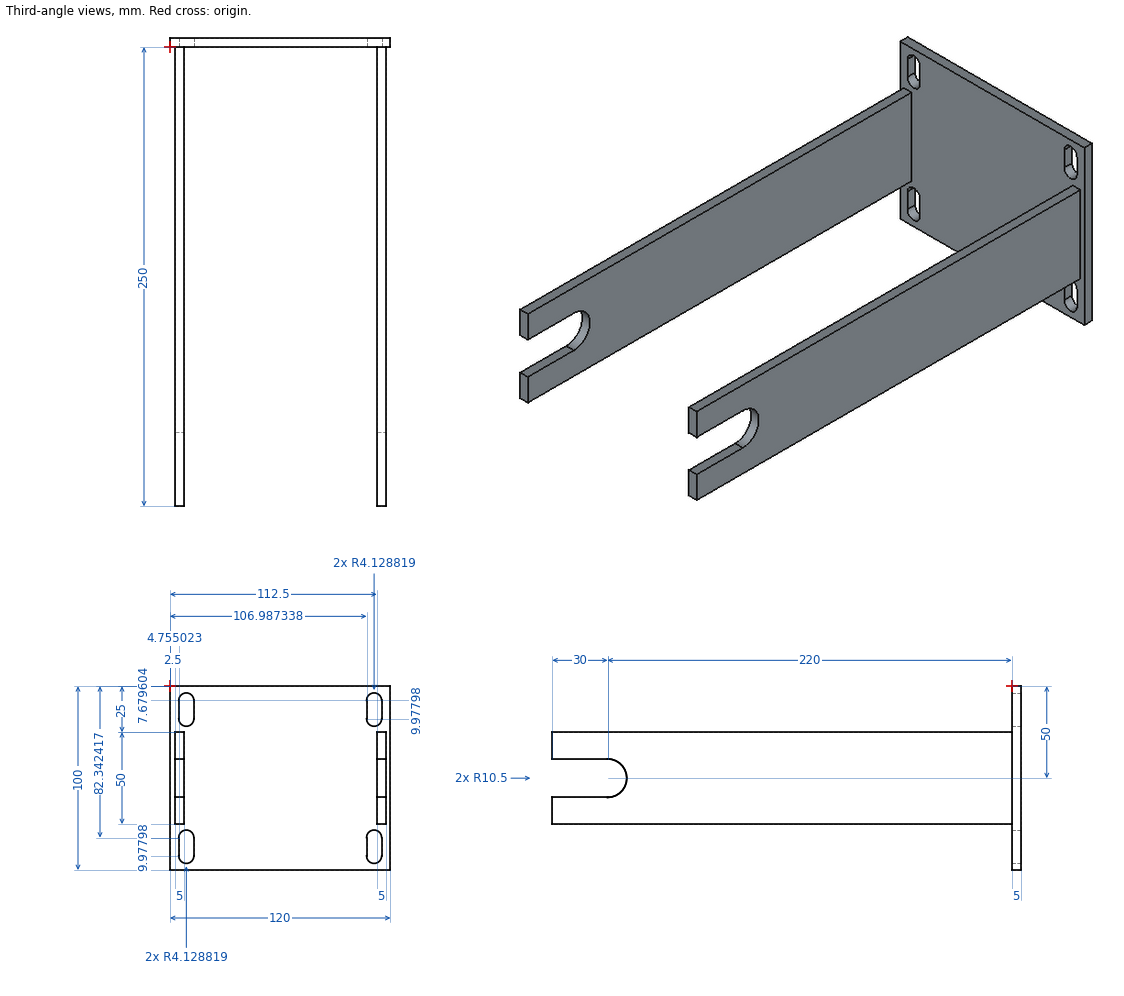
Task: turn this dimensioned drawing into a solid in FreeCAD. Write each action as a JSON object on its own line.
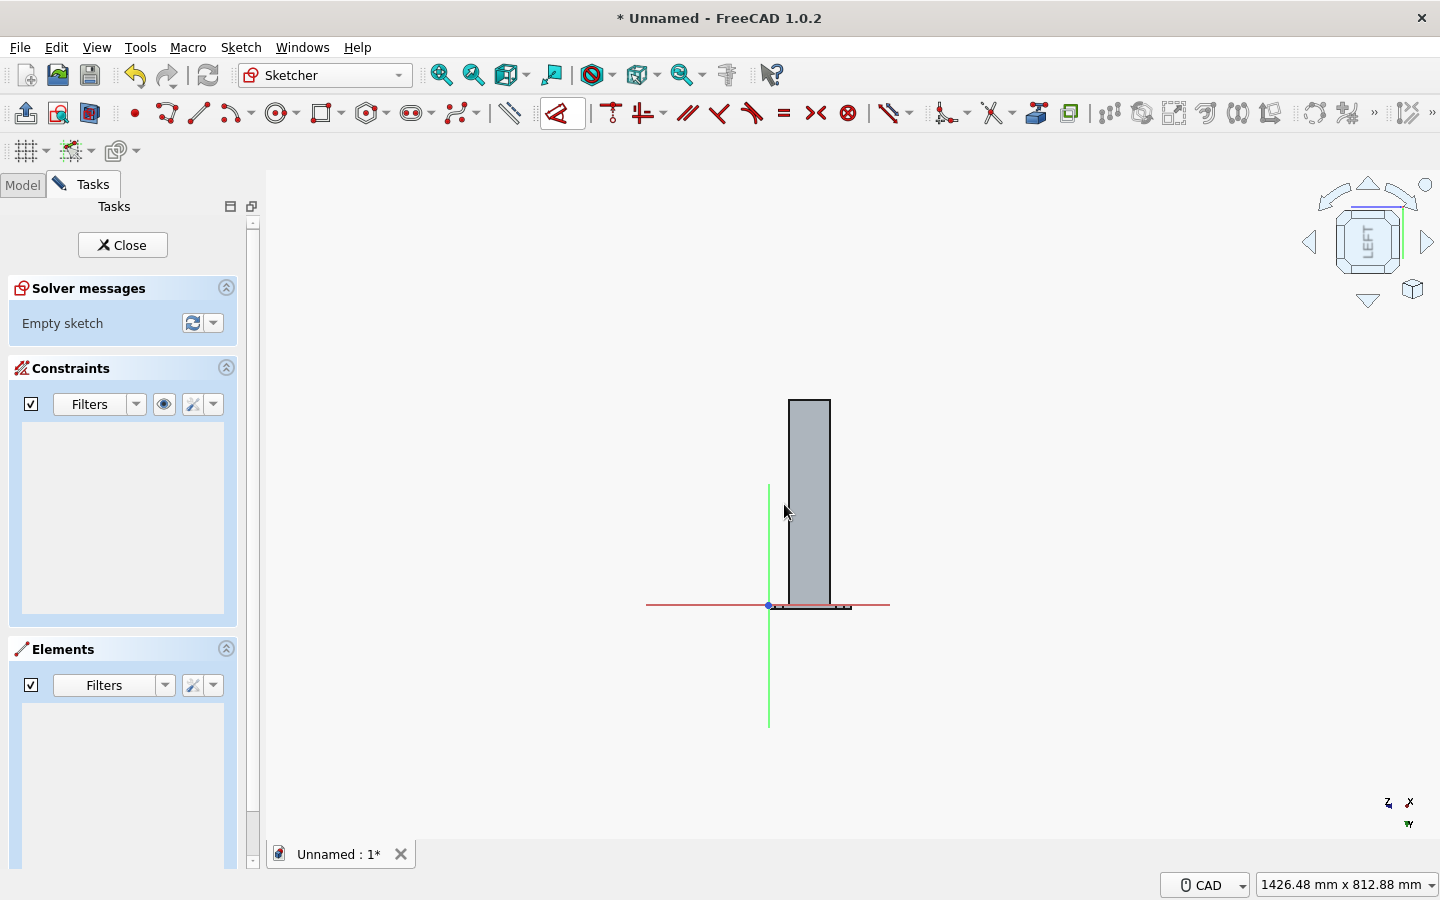
{"action": "scroll", "coordinate": [812, 403], "scroll_direction": "up", "scroll_amount": 12}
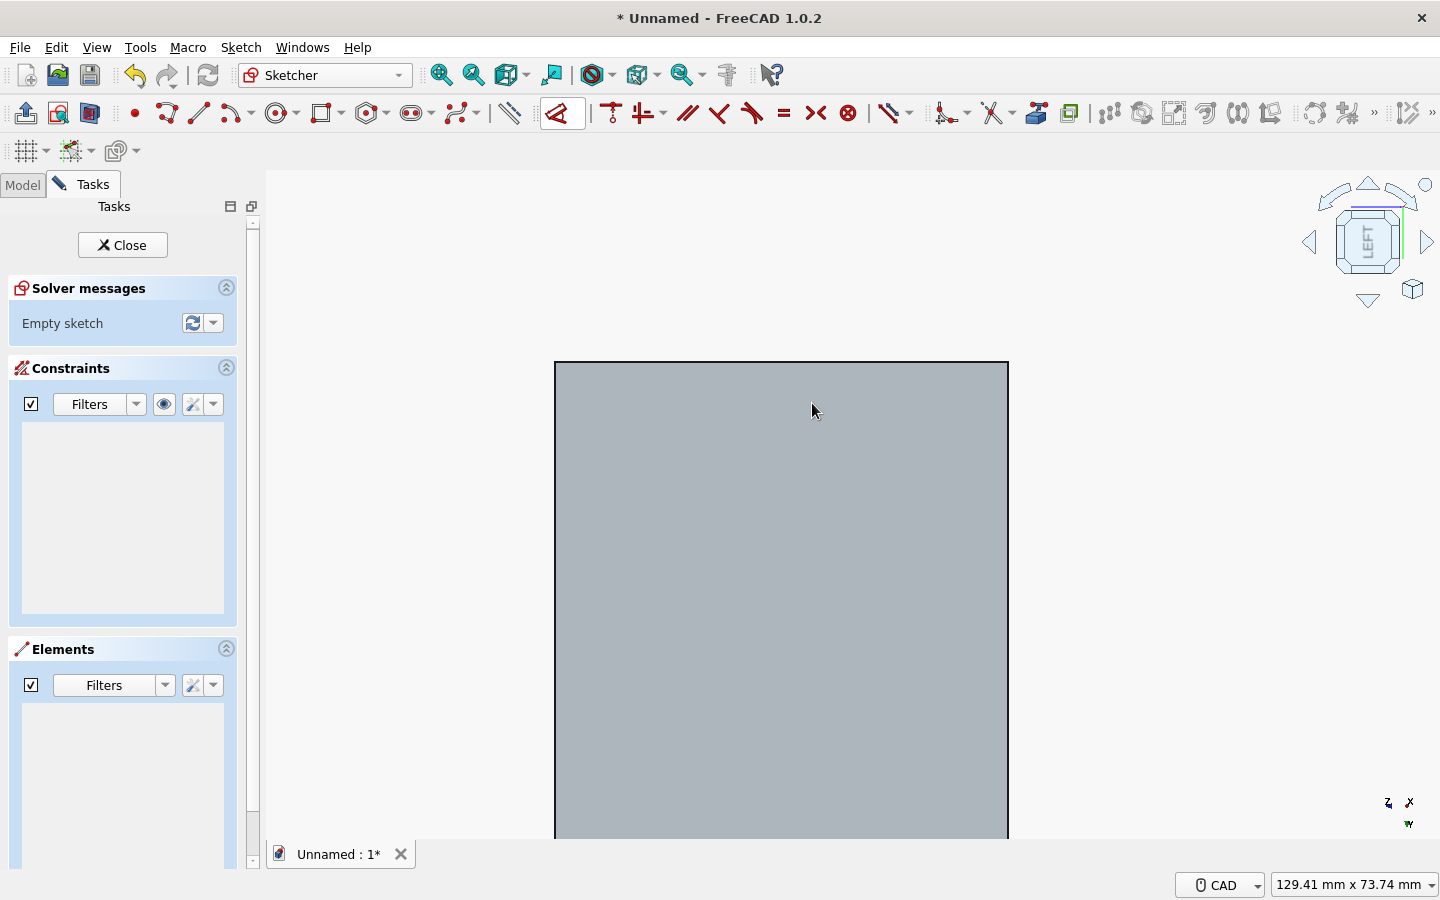
{"action": "left_click", "coordinate": [412, 114]}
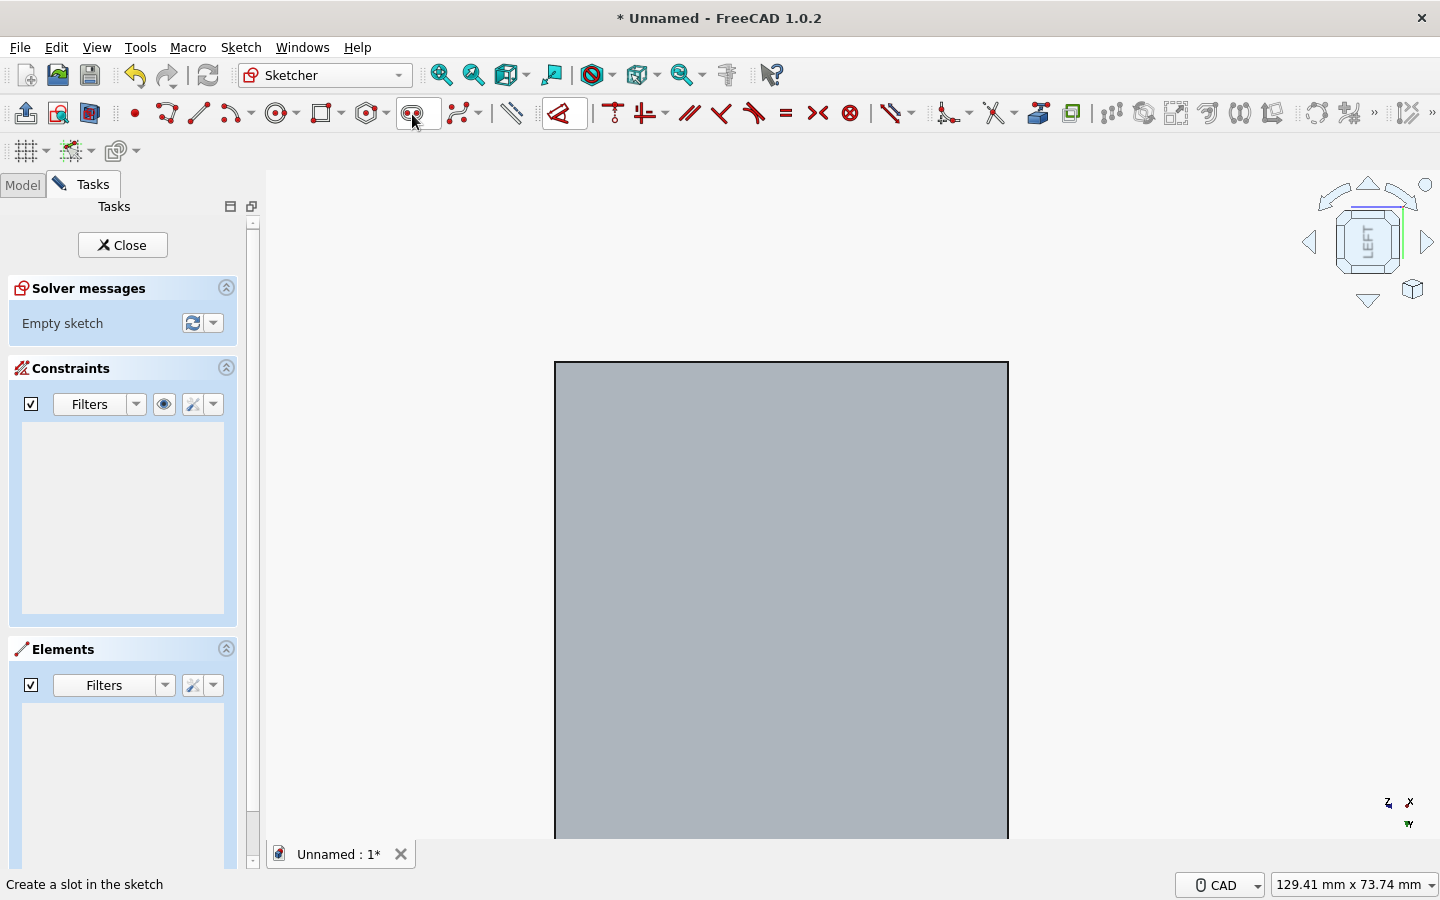
{"action": "left_click", "coordinate": [782, 634]}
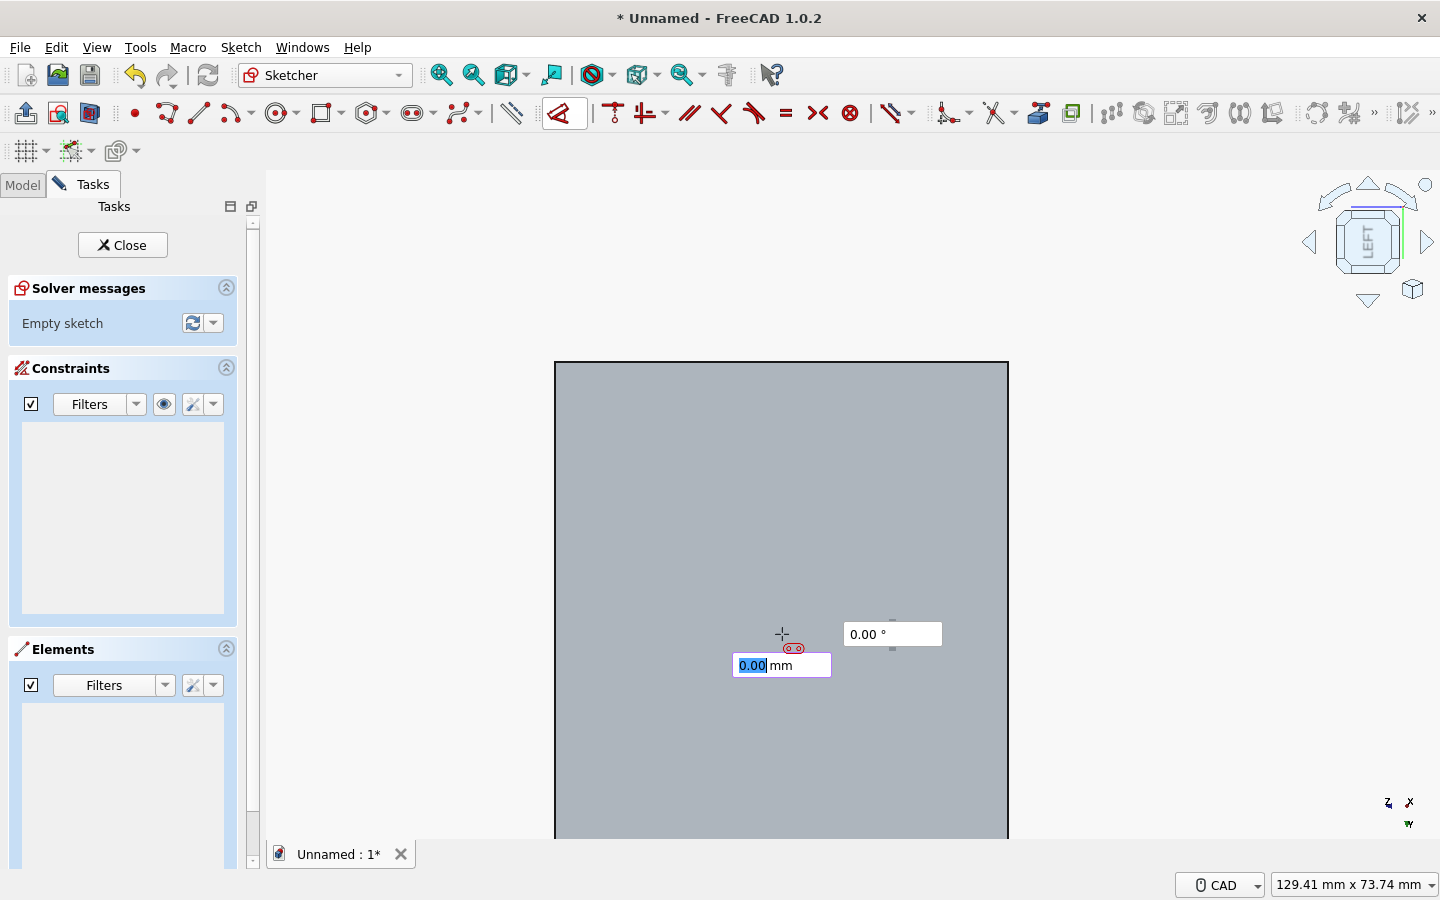
{"action": "left_click", "coordinate": [782, 362]}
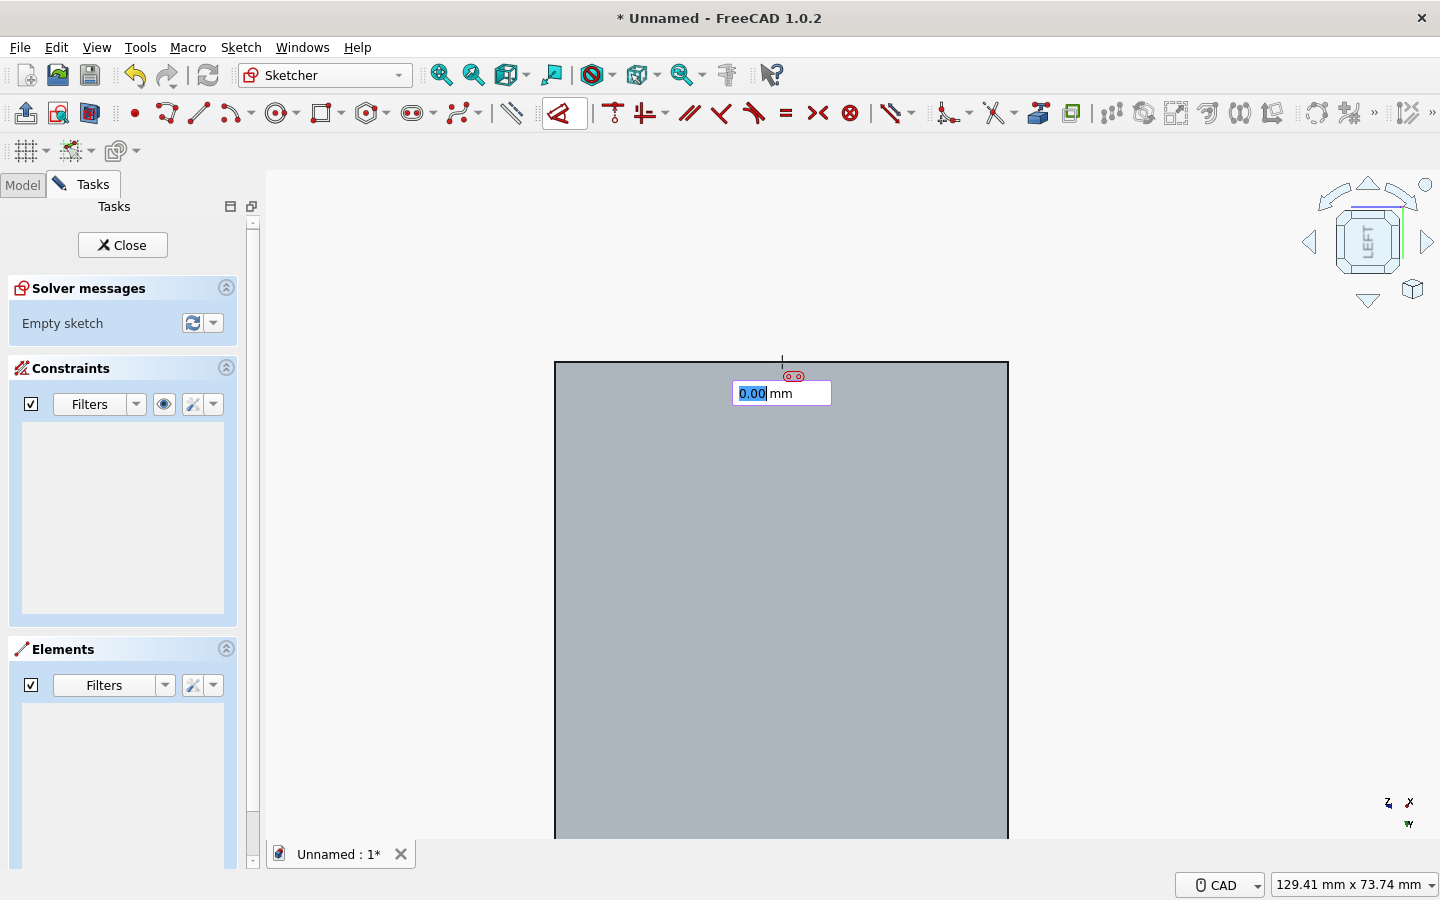
{"action": "left_click", "coordinate": [877, 498]}
{"action": "key", "text": "Escape"}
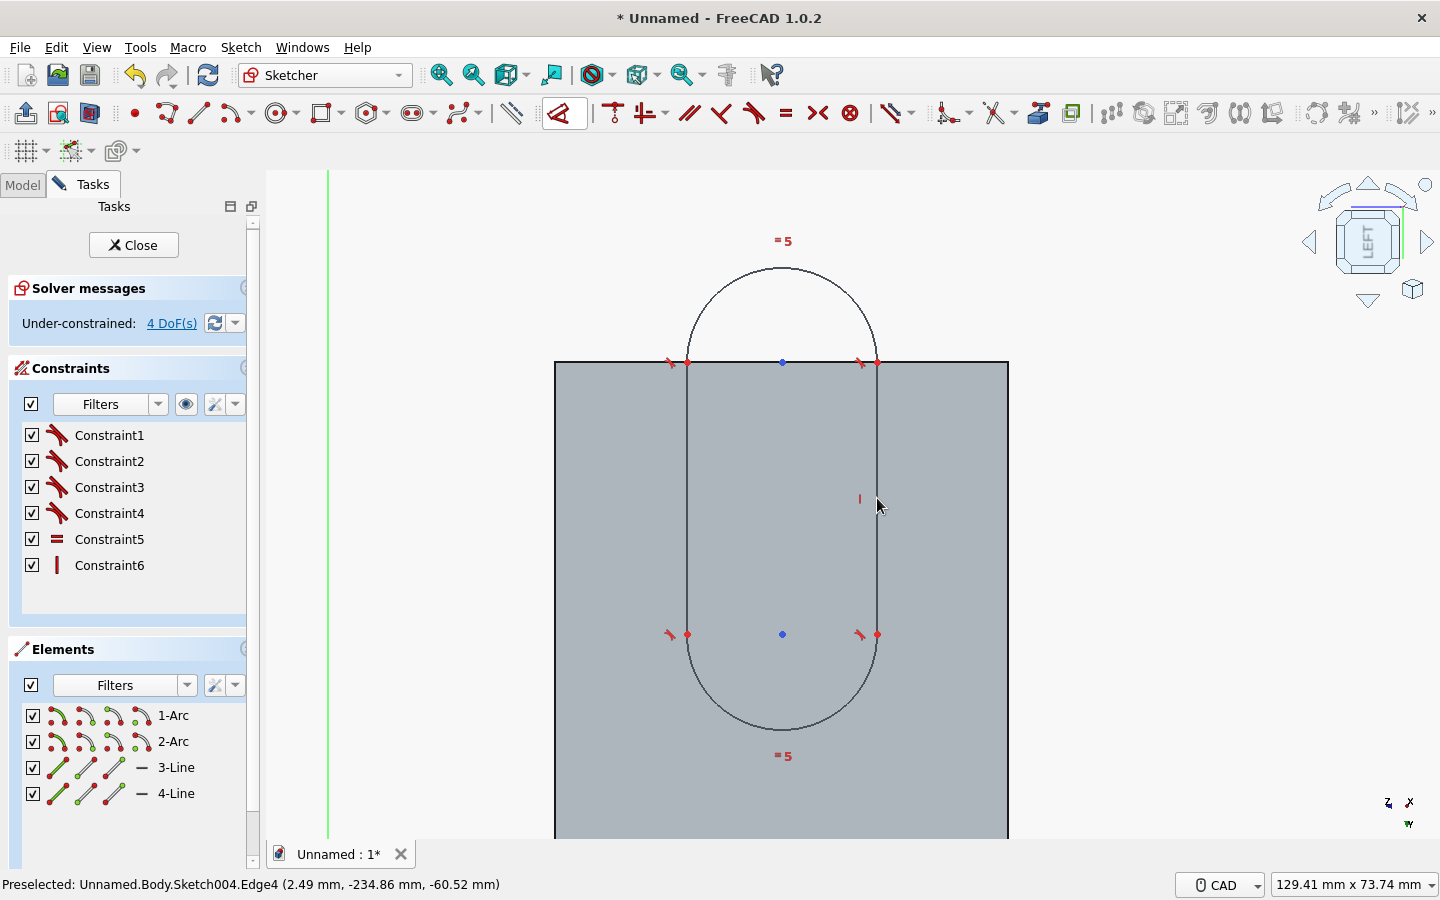
{"action": "left_click", "coordinate": [726, 712]}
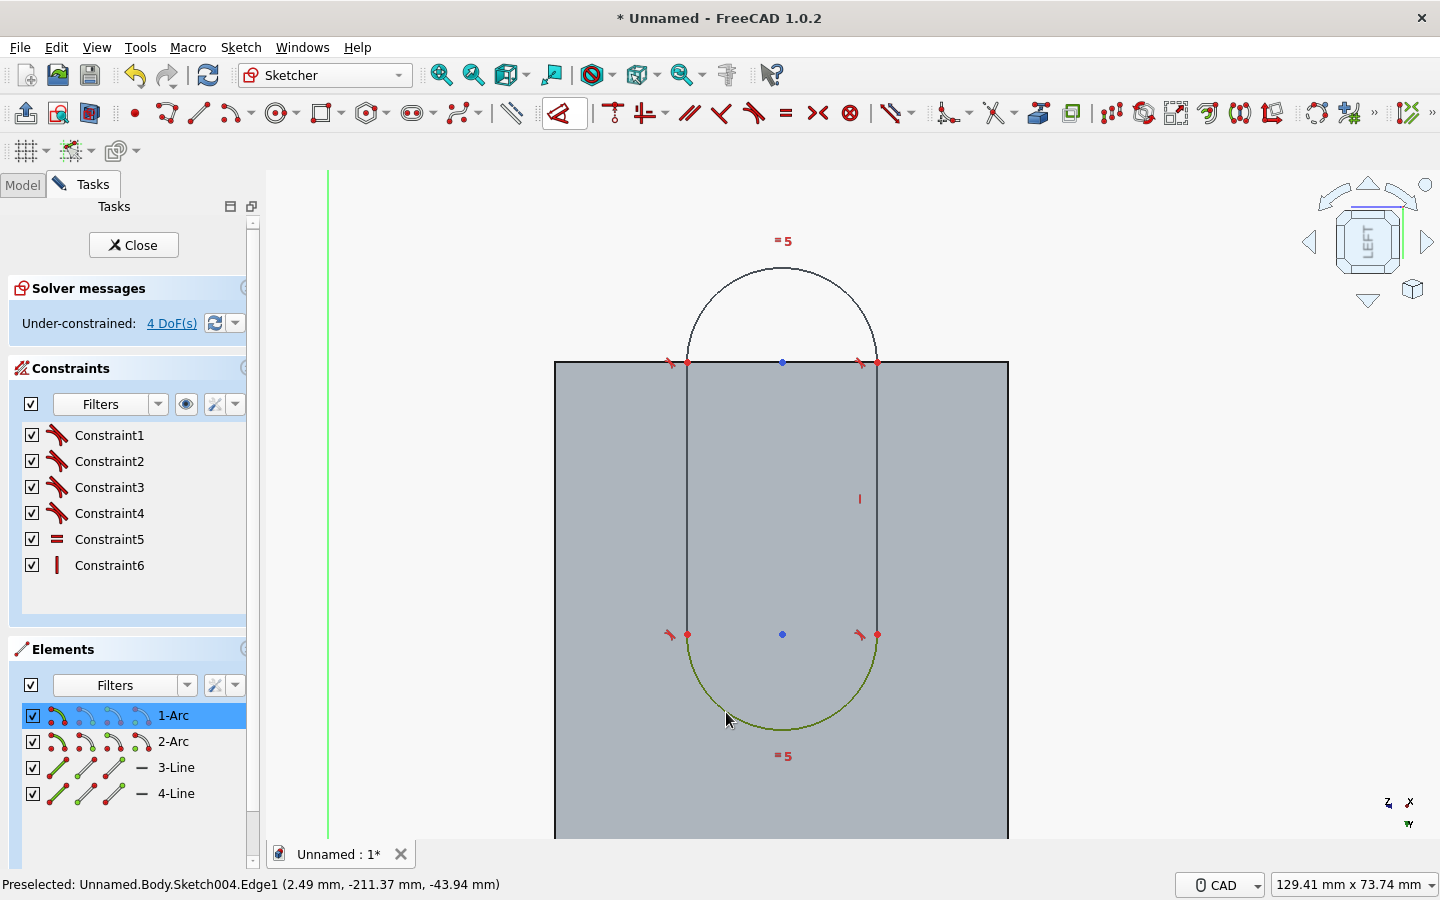
{"action": "key", "text": "k r"}